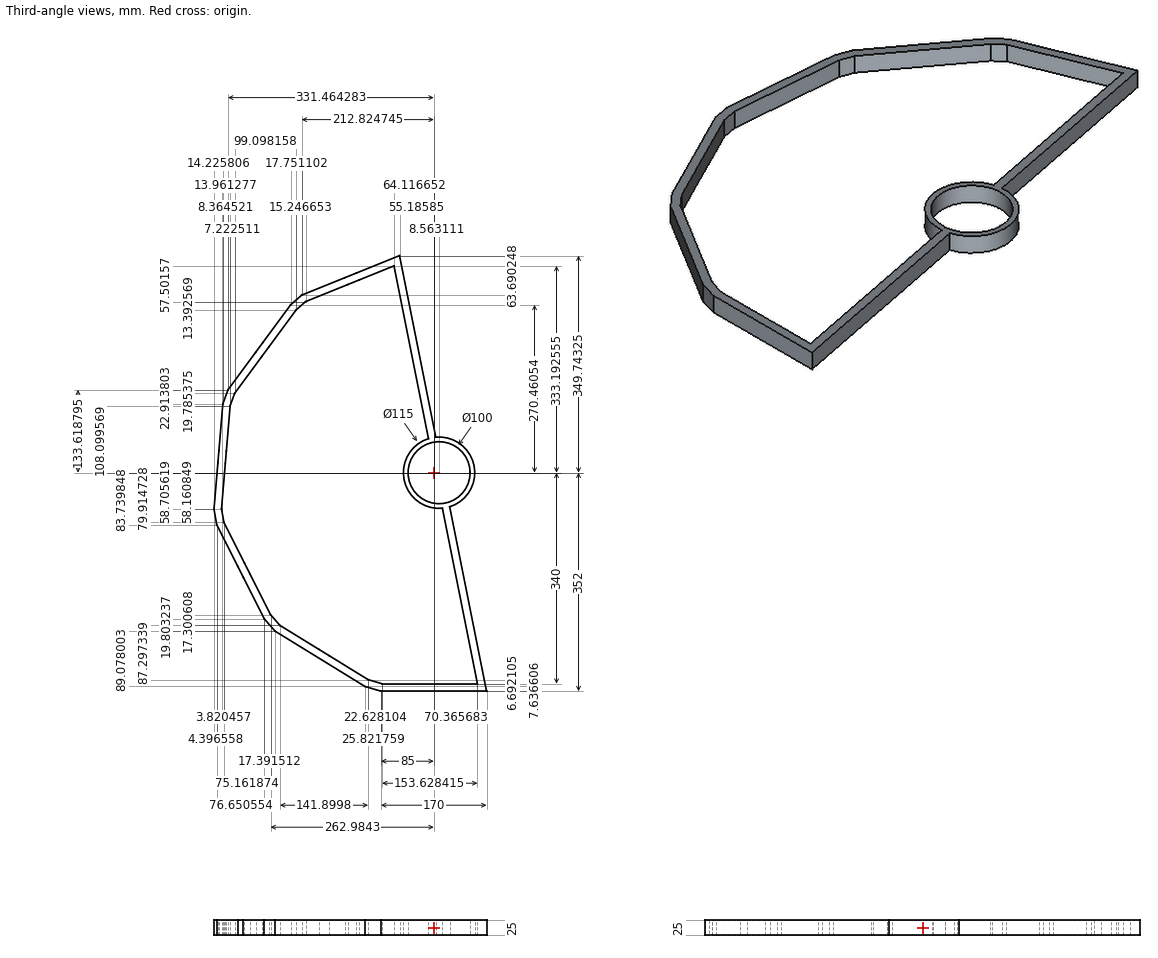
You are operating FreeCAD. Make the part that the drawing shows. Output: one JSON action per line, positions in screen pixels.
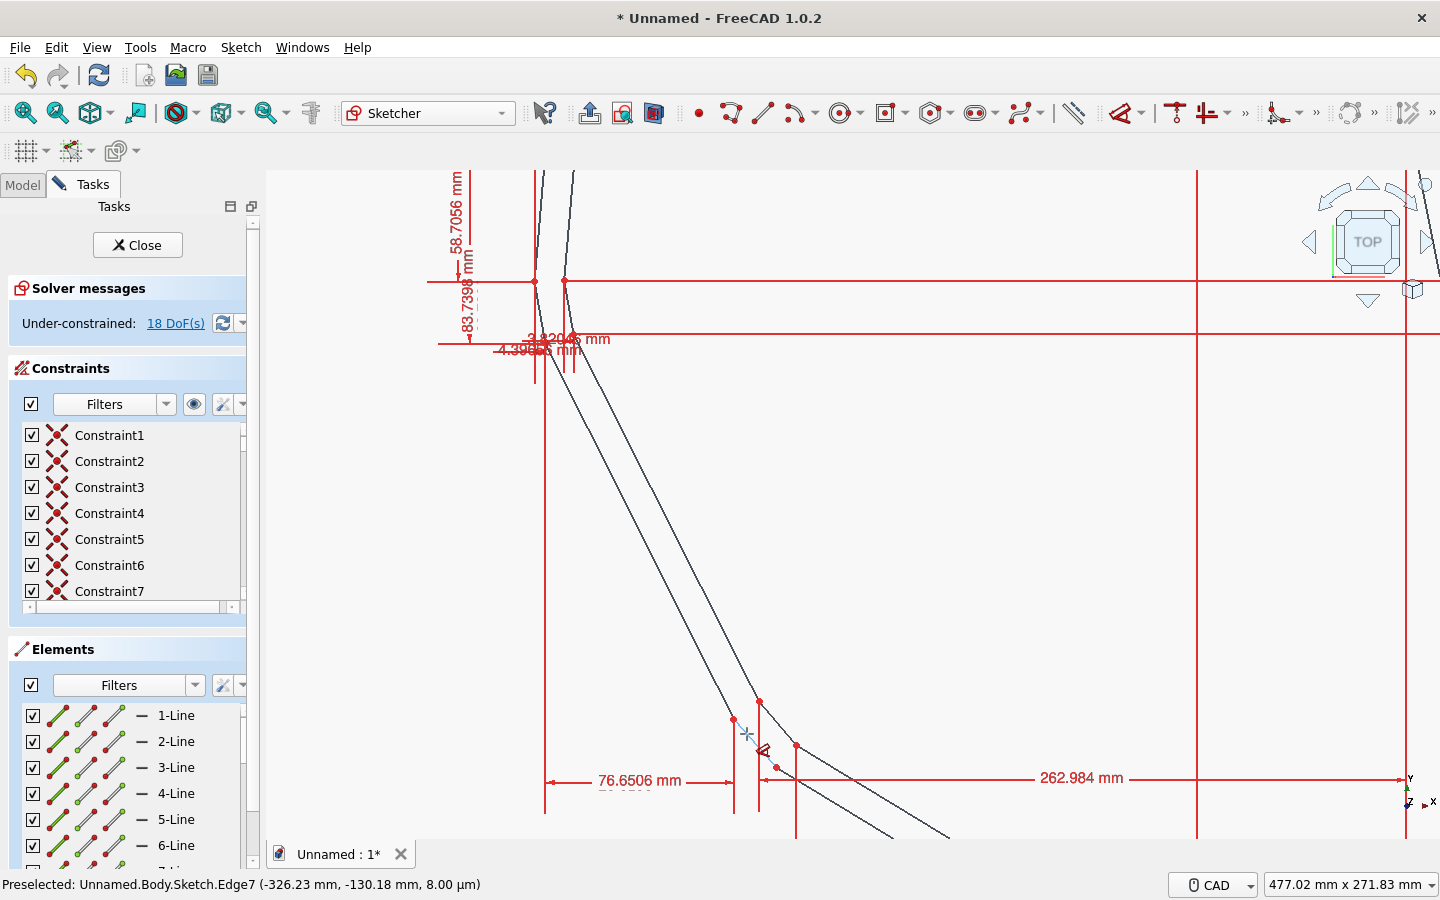
{"action": "left_click", "coordinate": [747, 734]}
{"action": "left_click", "coordinate": [755, 802]}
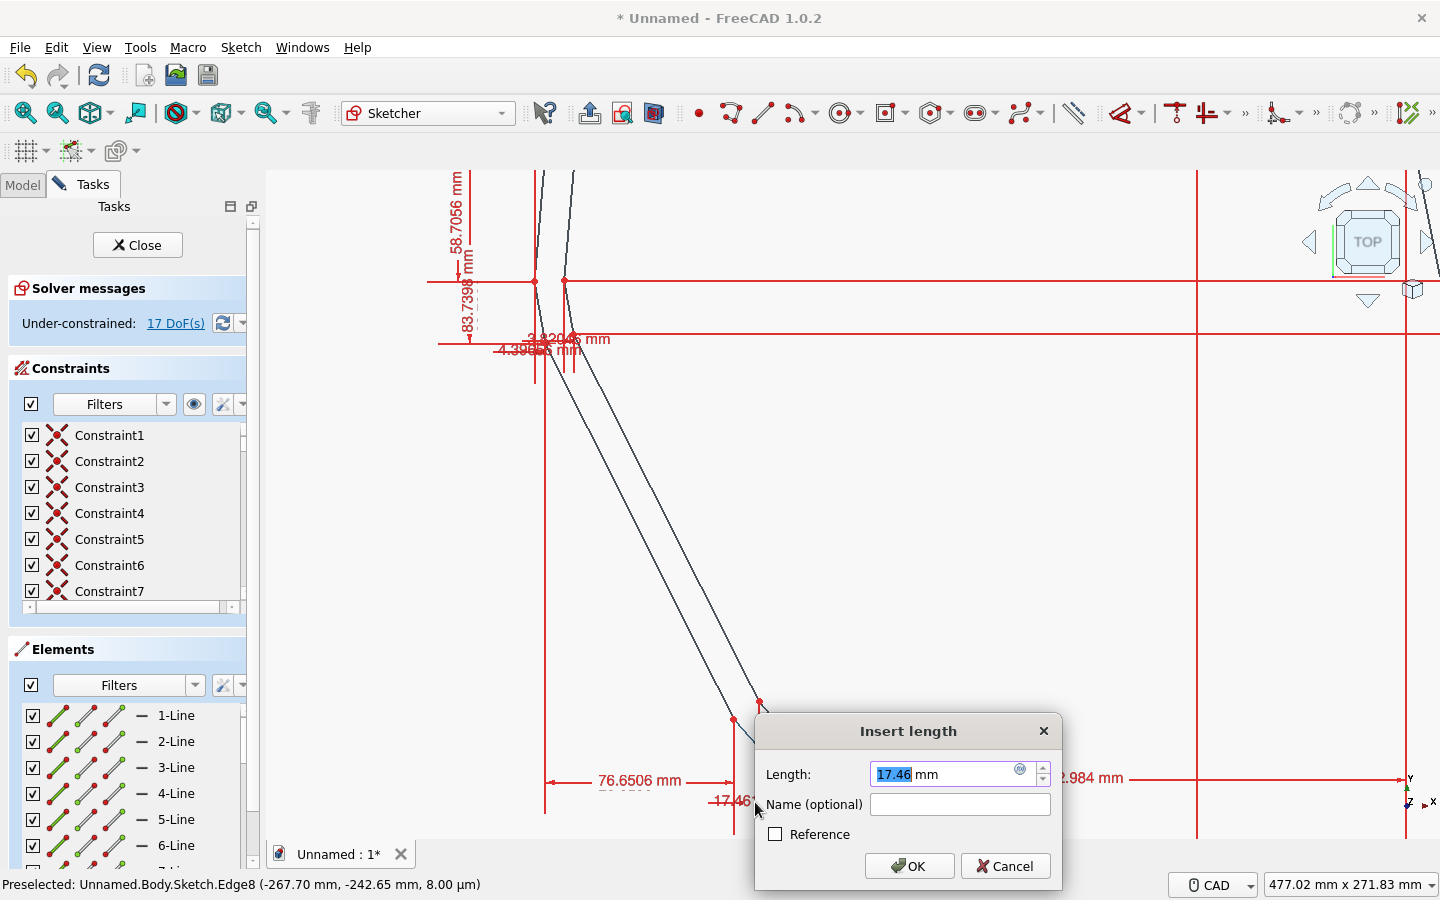
{"action": "type", "text": "17.391512"}
{"action": "key", "text": "Return"}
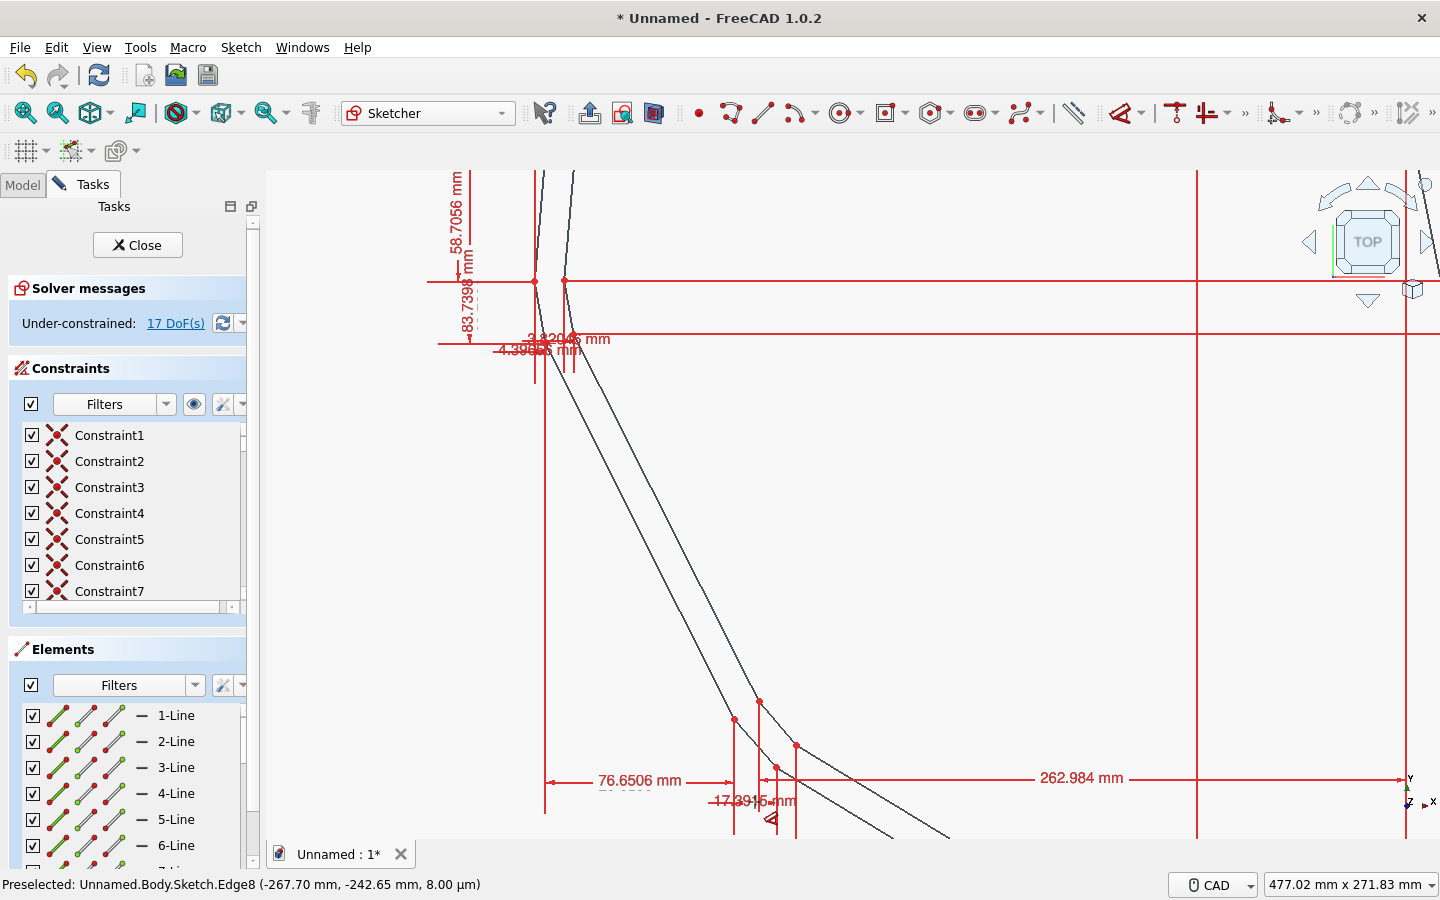
{"action": "left_click", "coordinate": [747, 734]}
{"action": "left_click", "coordinate": [700, 744]}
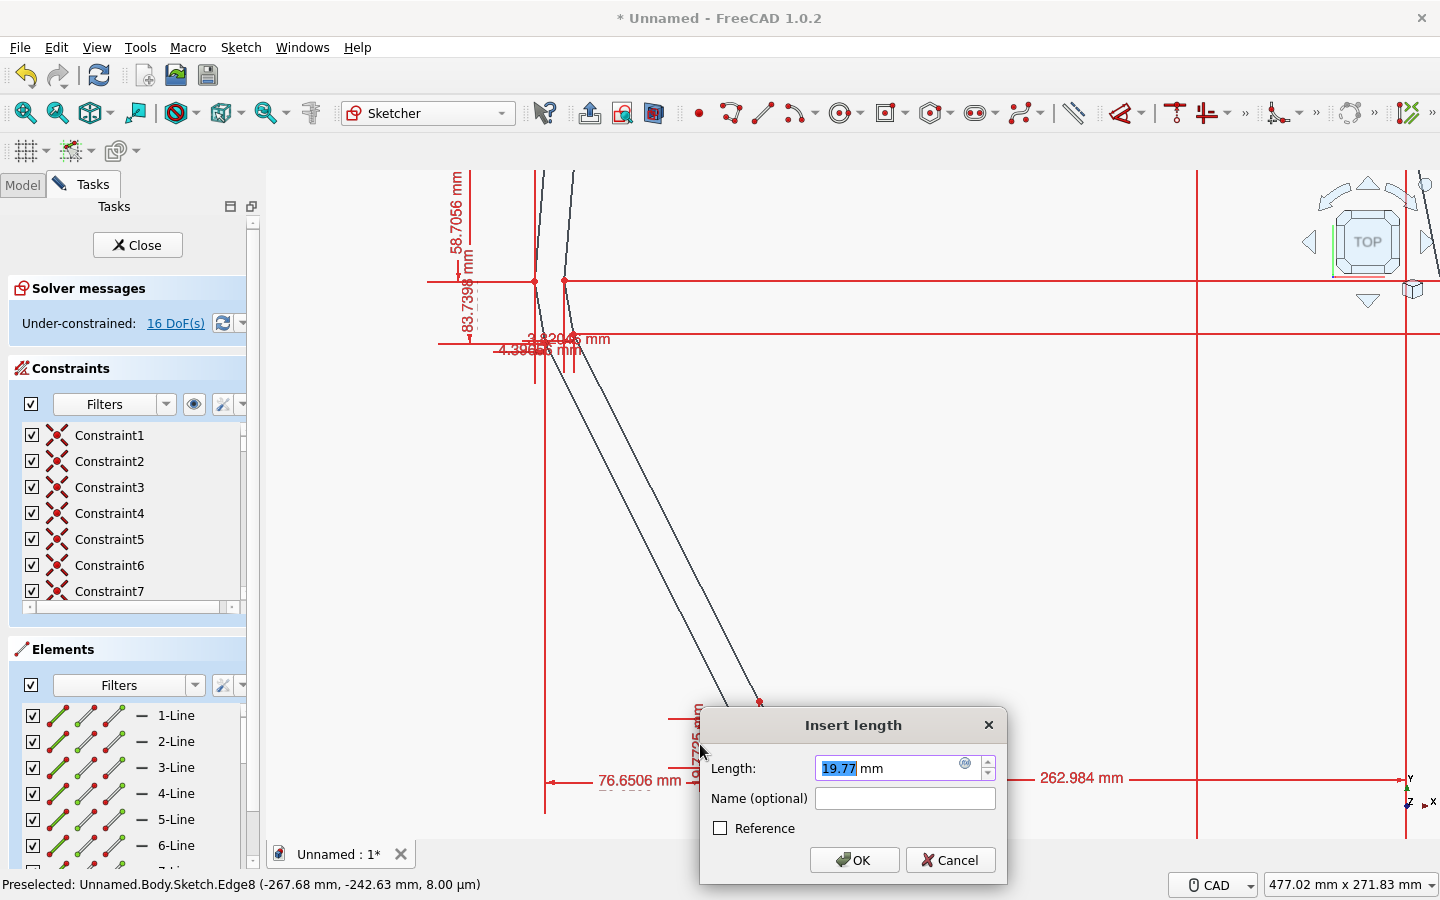
{"action": "type", "text": "19.803237"}
{"action": "key", "text": "Return"}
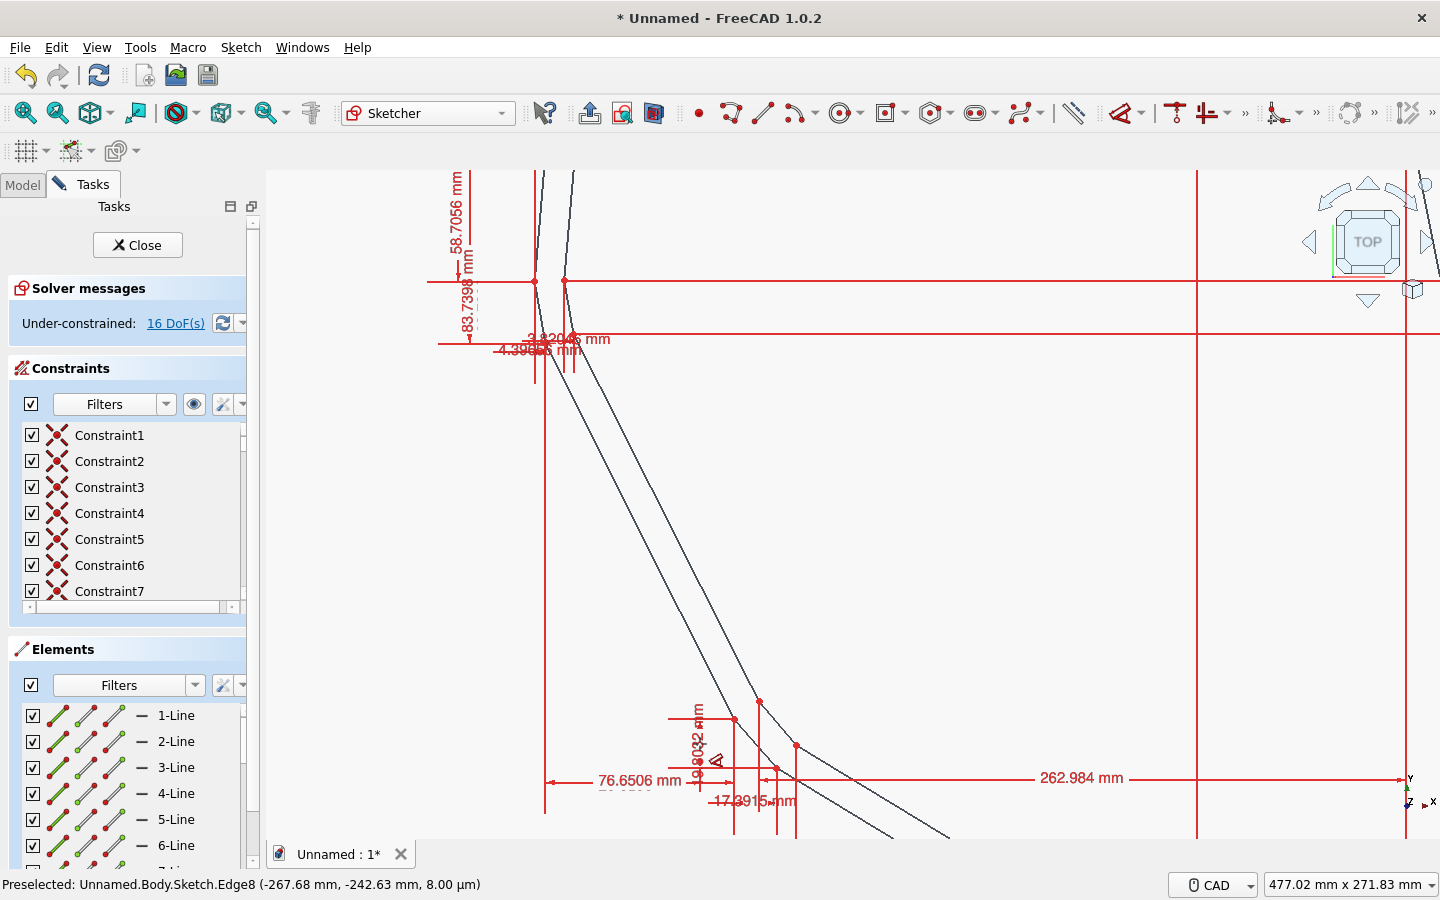
{"action": "scroll", "coordinate": [689, 624], "scroll_direction": "down", "scroll_amount": 7}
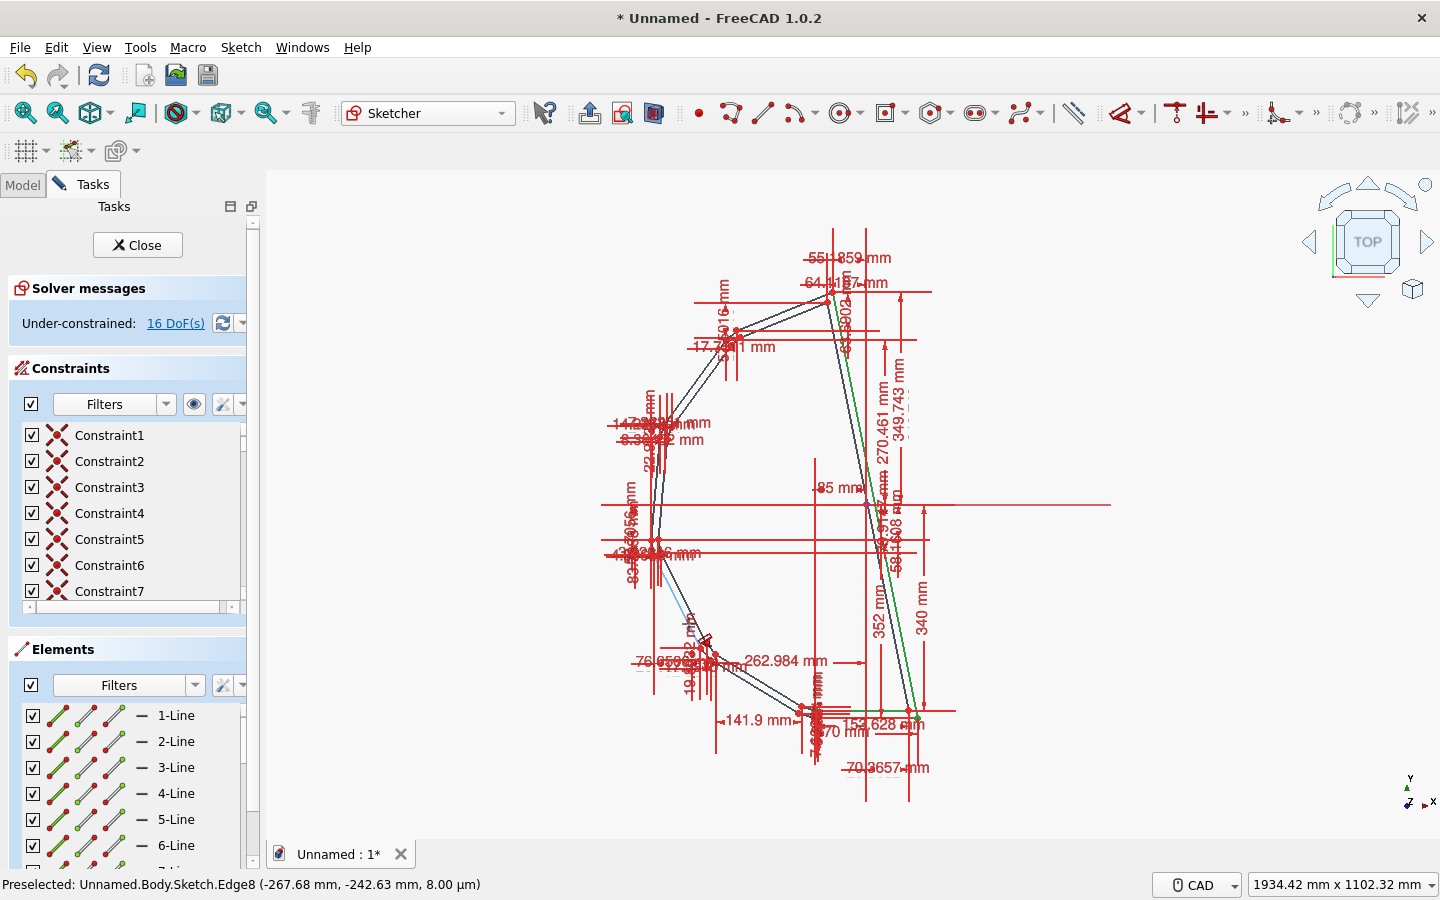
{"action": "scroll", "coordinate": [737, 676], "scroll_direction": "up", "scroll_amount": 4}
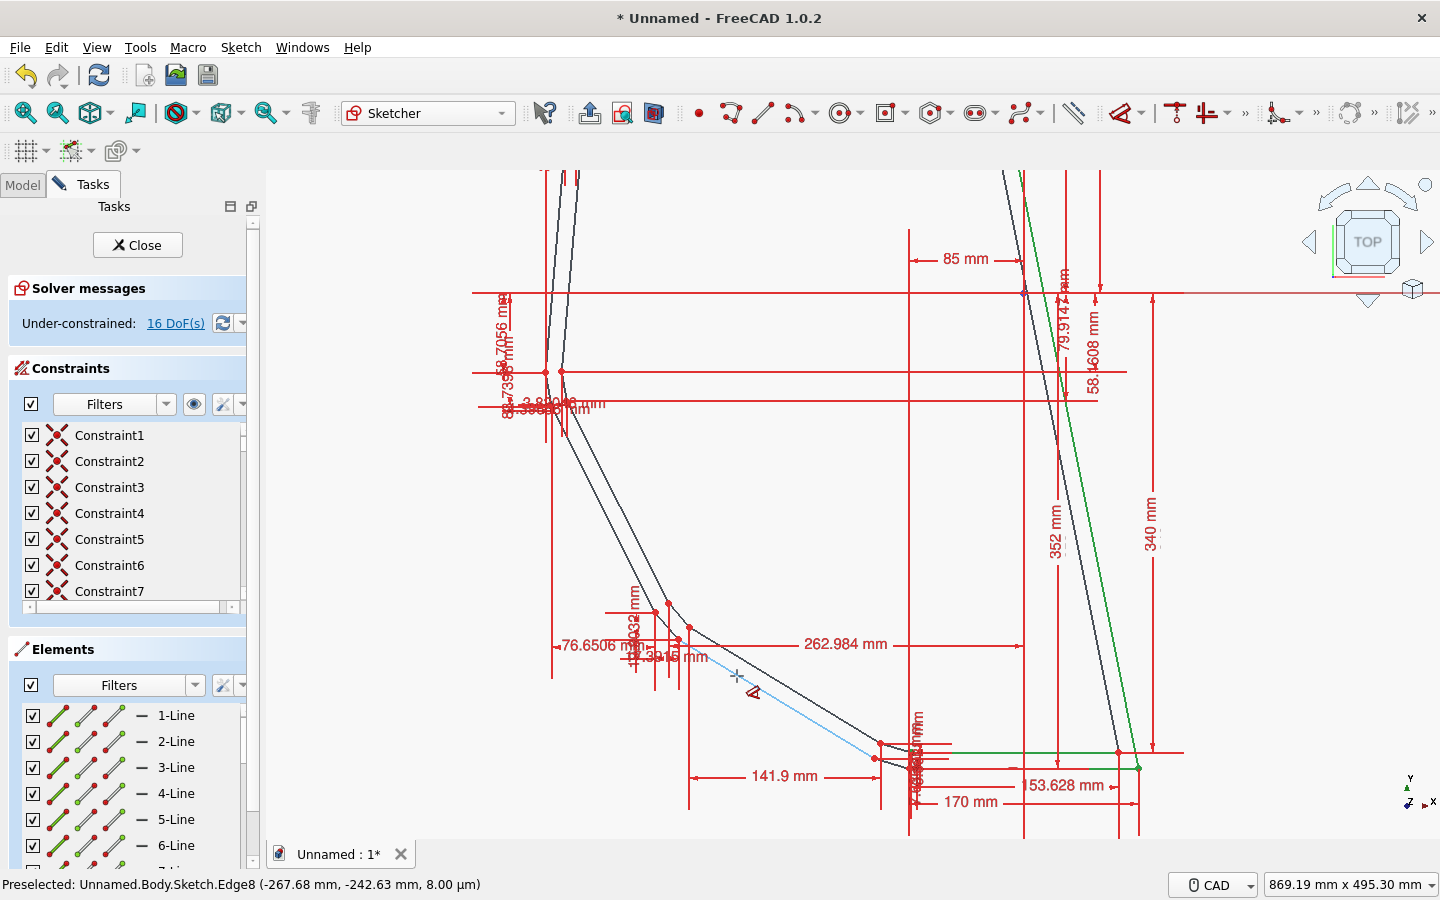
{"action": "left_click", "coordinate": [737, 675]}
{"action": "left_click", "coordinate": [645, 699]}